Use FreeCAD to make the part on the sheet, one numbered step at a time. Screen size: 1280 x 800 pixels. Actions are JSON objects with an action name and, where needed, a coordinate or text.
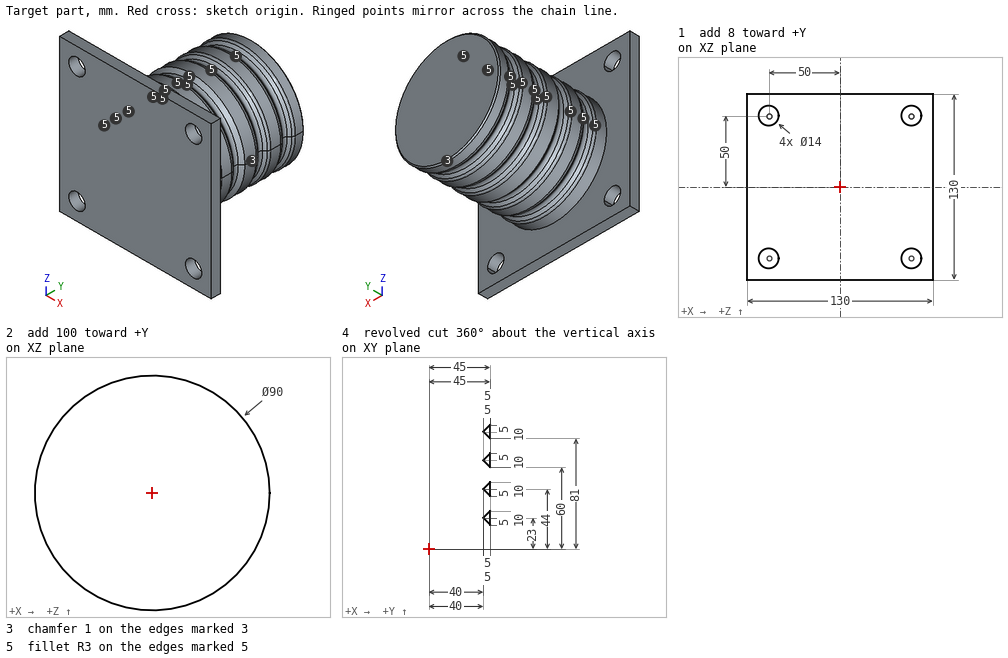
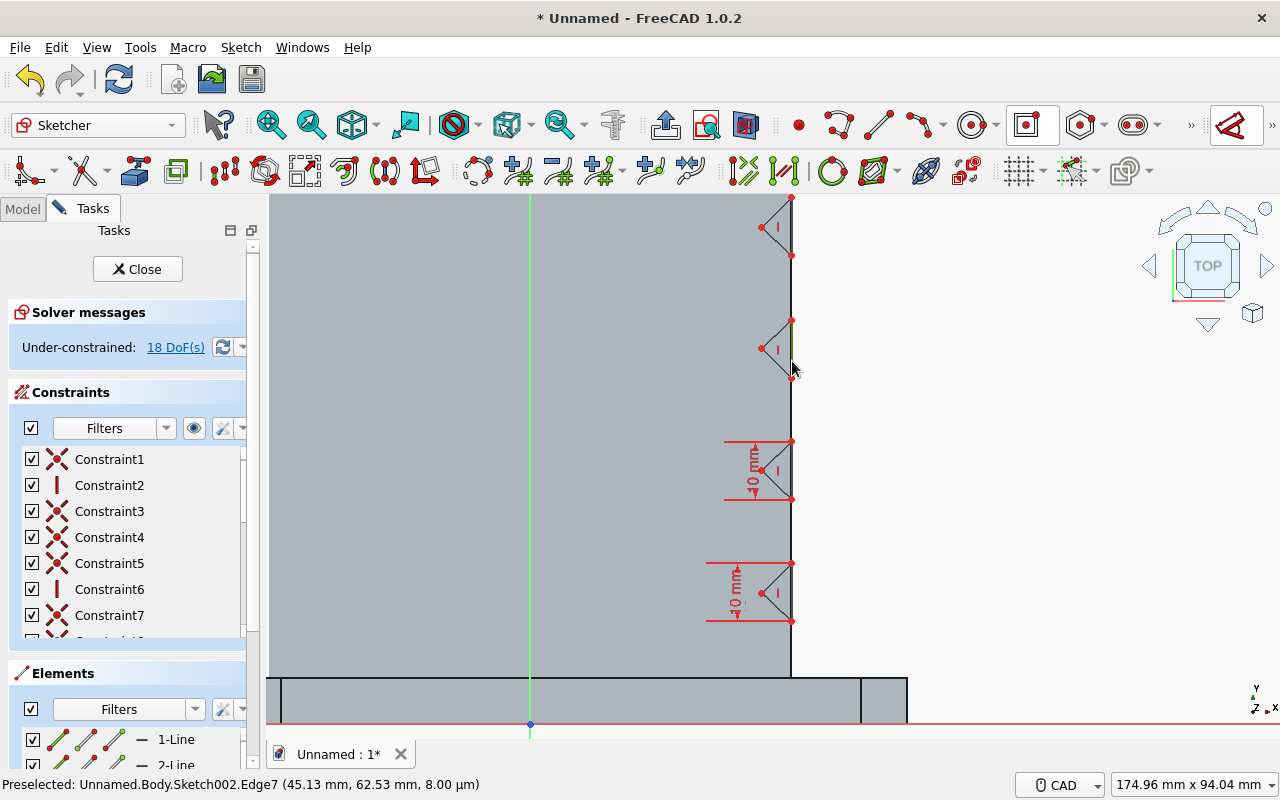
{"action": "key", "text": "i"}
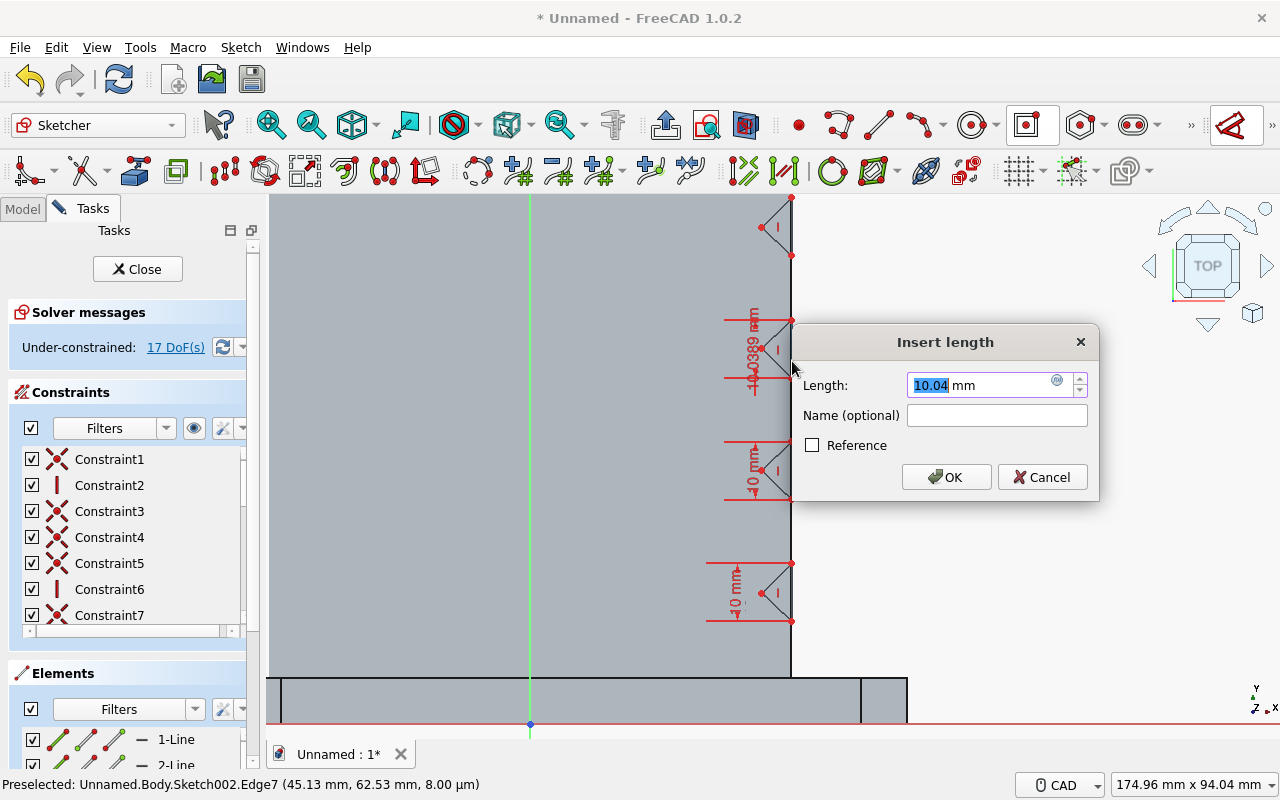
{"action": "type", "text": "10"}
{"action": "key", "text": "Return"}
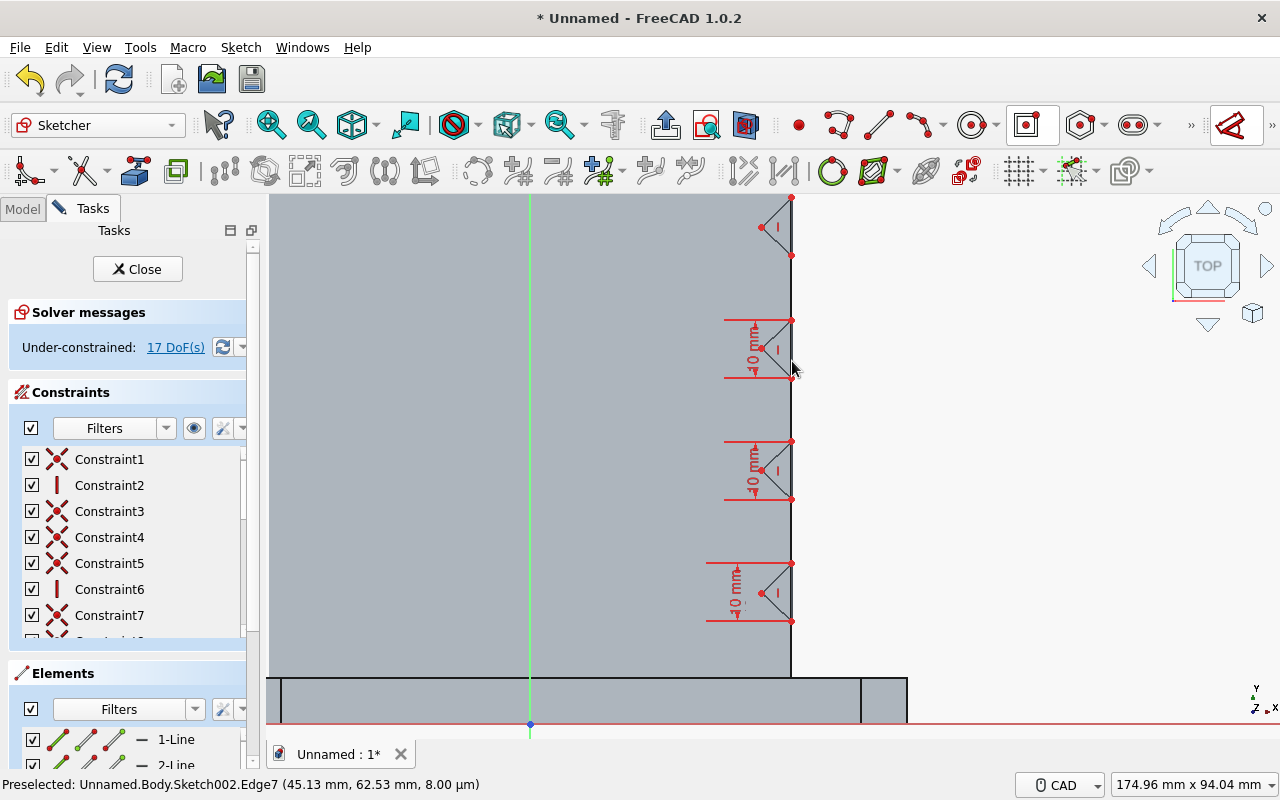
{"action": "left_click", "coordinate": [792, 238]}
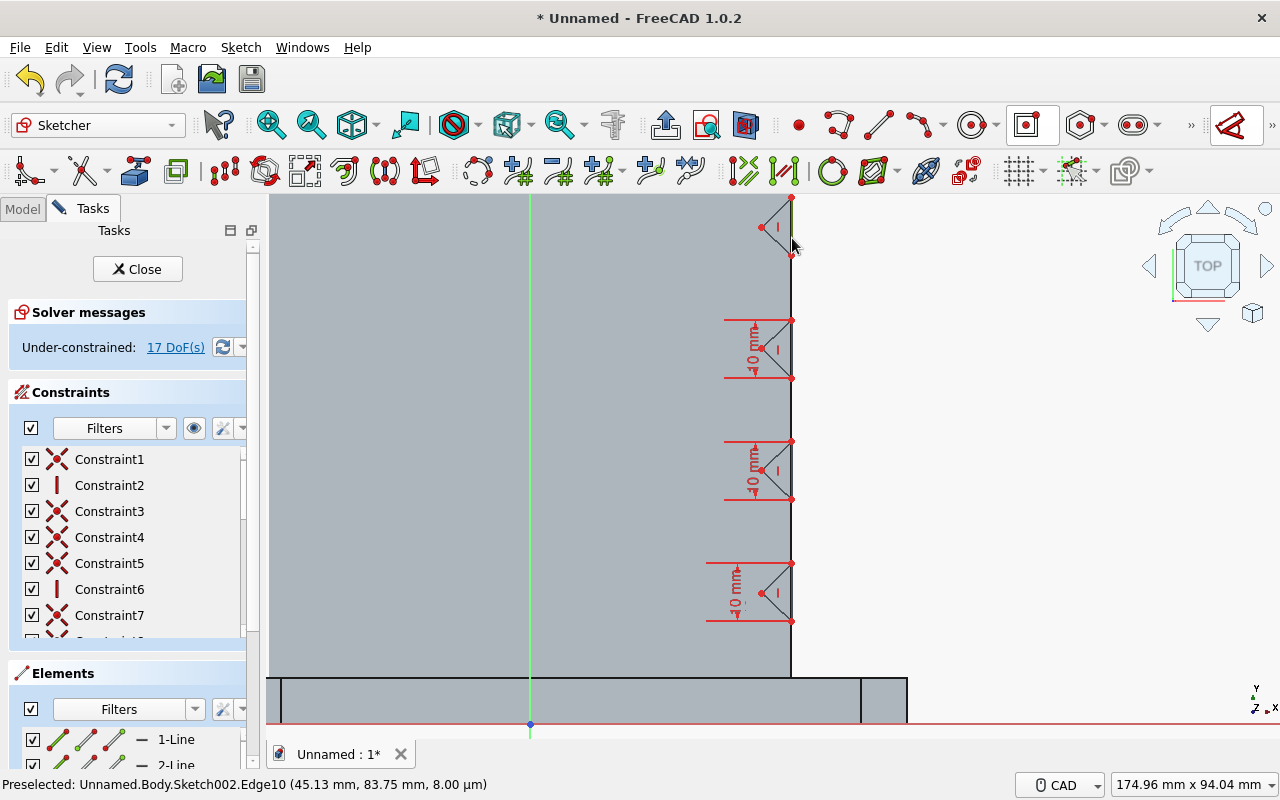
{"action": "key", "text": "i"}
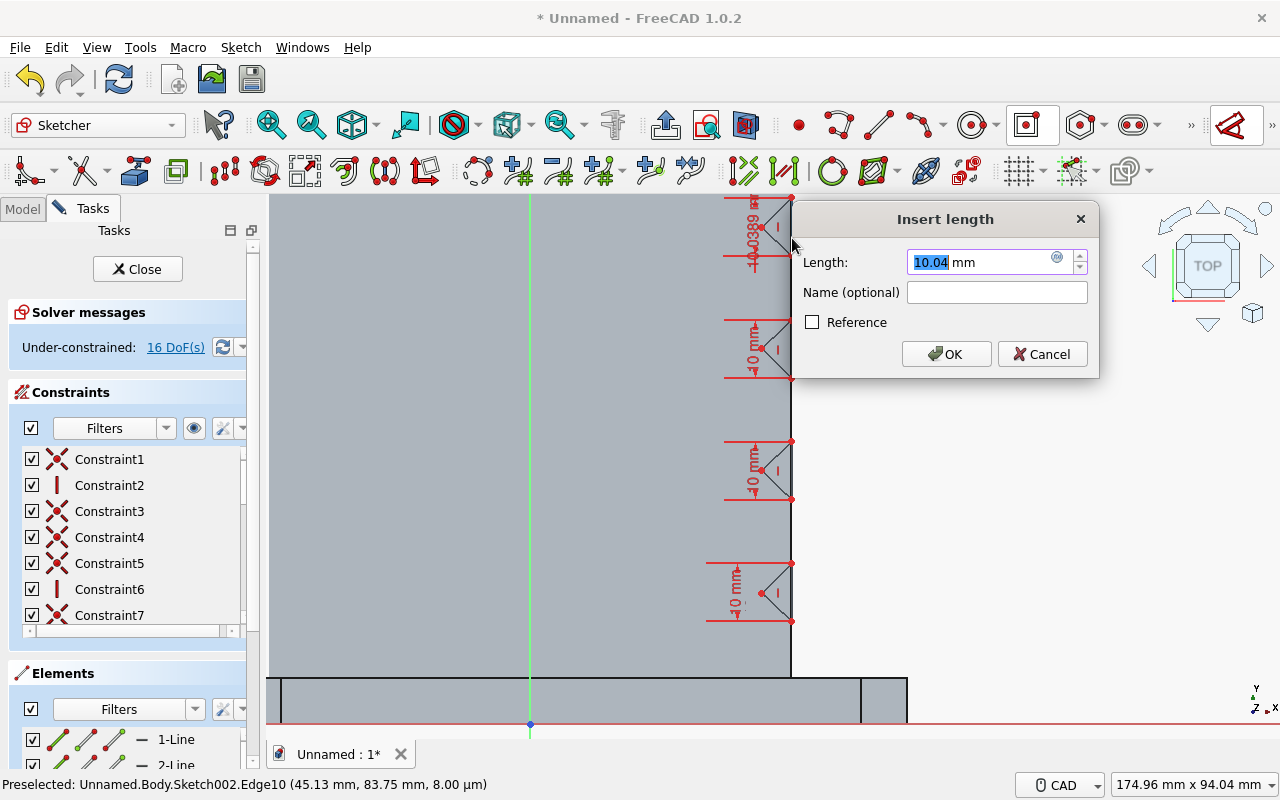
{"action": "type", "text": "10"}
{"action": "key", "text": "Return"}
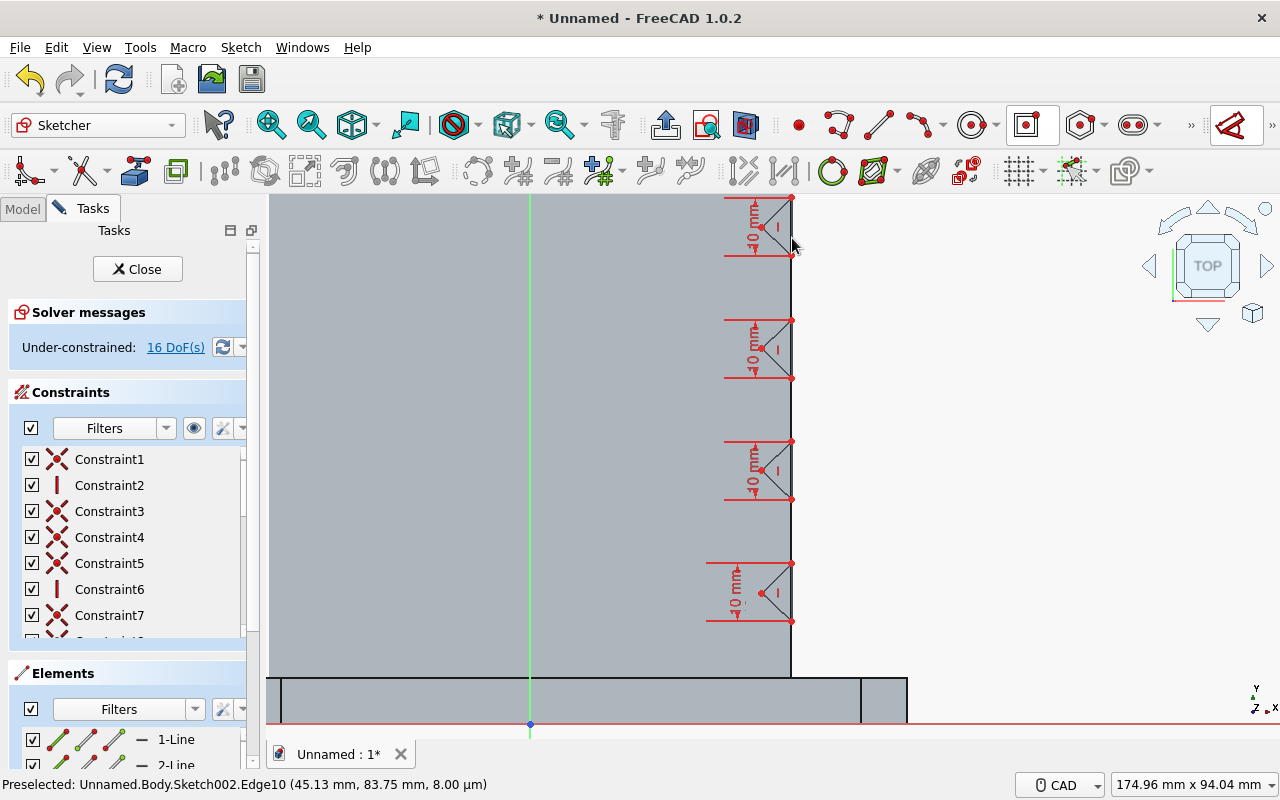
{"action": "scroll", "coordinate": [771, 602], "scroll_direction": "up", "scroll_amount": 2}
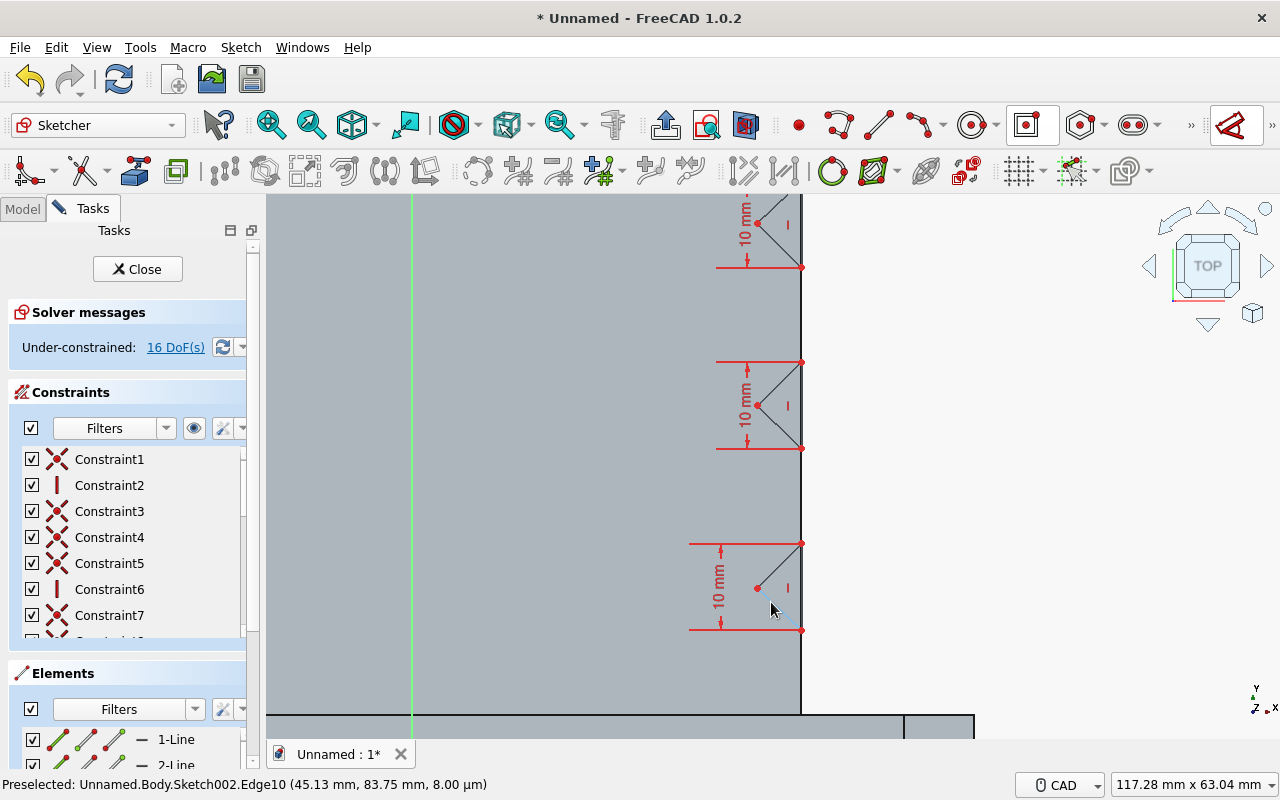
{"action": "left_click", "coordinate": [771, 601]}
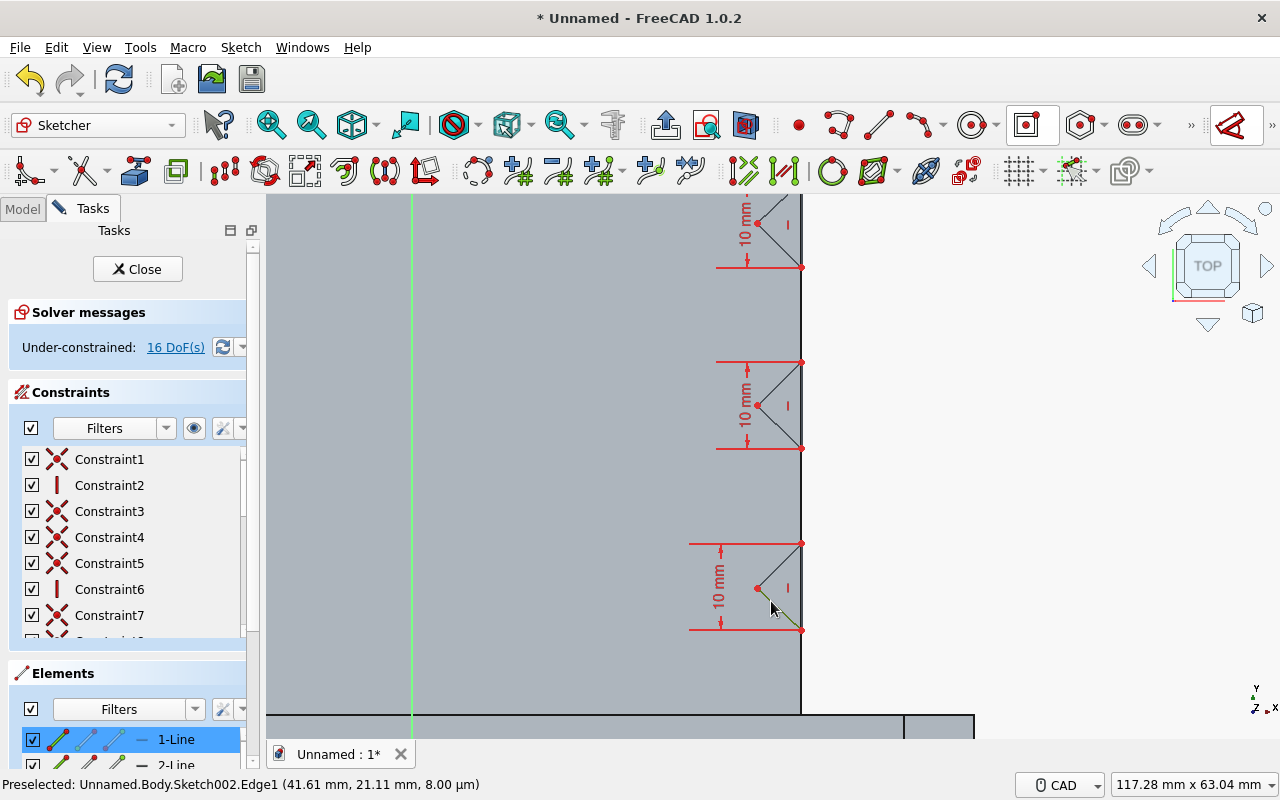
{"action": "key", "text": "l"}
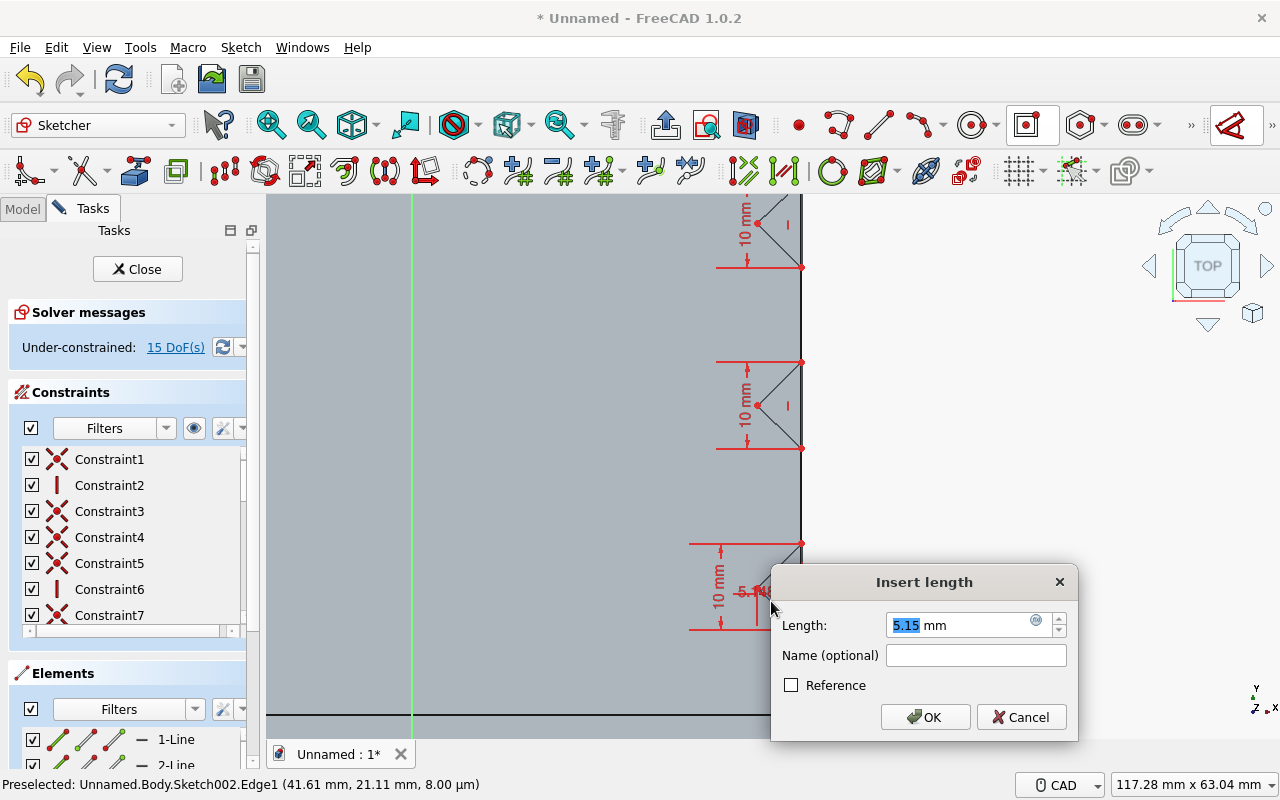
{"action": "type", "text": "5"}
{"action": "key", "text": "Return"}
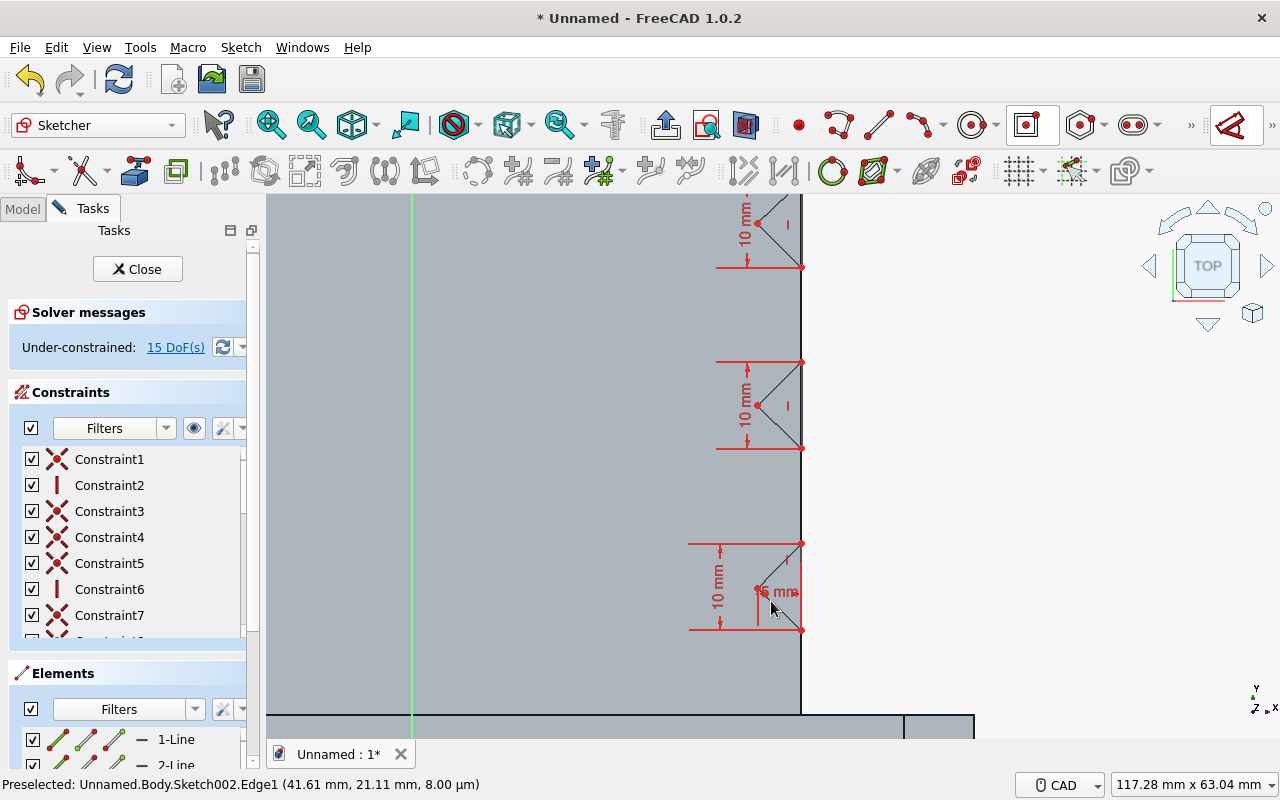
{"action": "left_click", "coordinate": [771, 601]}